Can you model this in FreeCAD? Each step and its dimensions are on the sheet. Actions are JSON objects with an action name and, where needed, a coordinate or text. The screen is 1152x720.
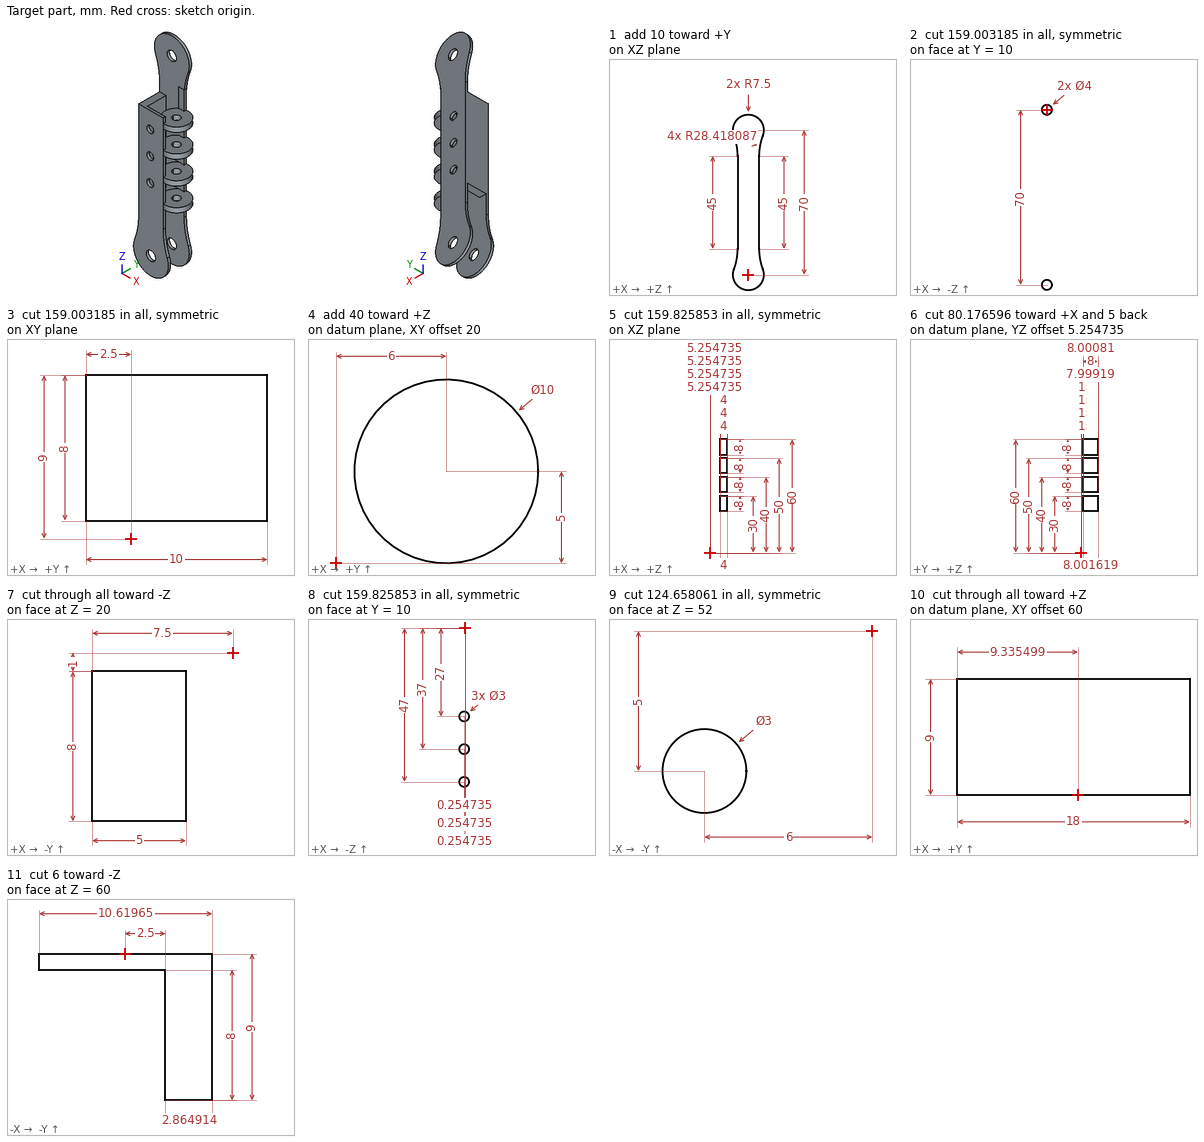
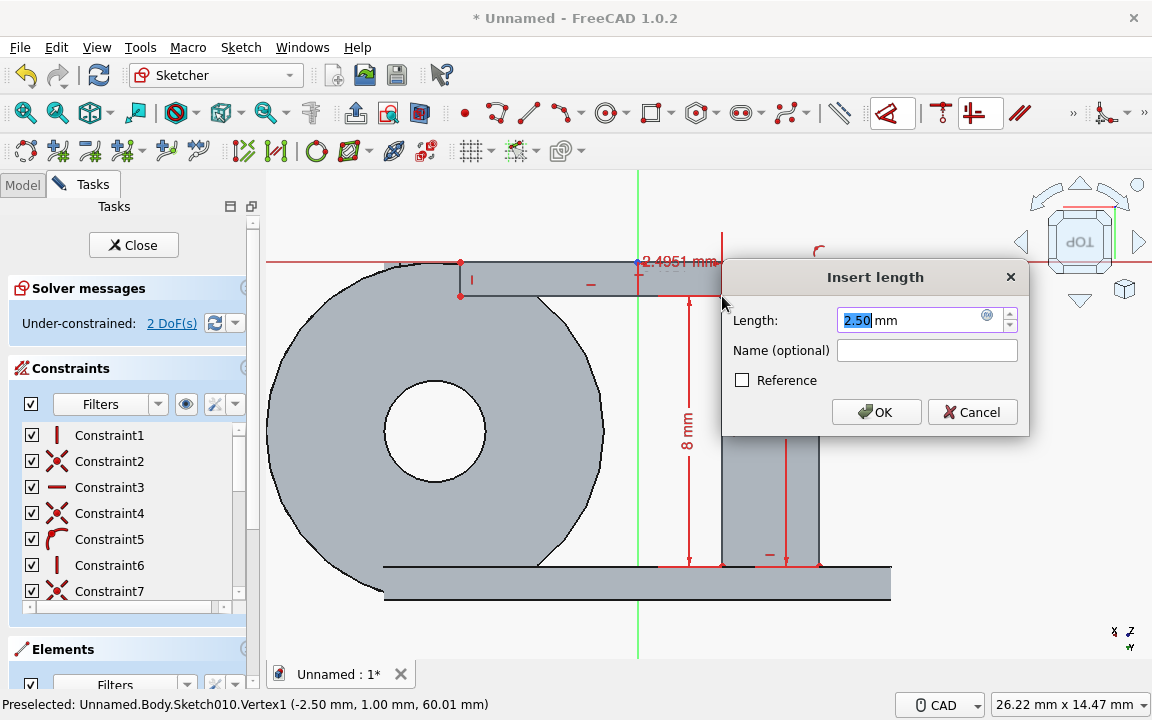
{"action": "type", "text": "2.5"}
{"action": "key", "text": "Return"}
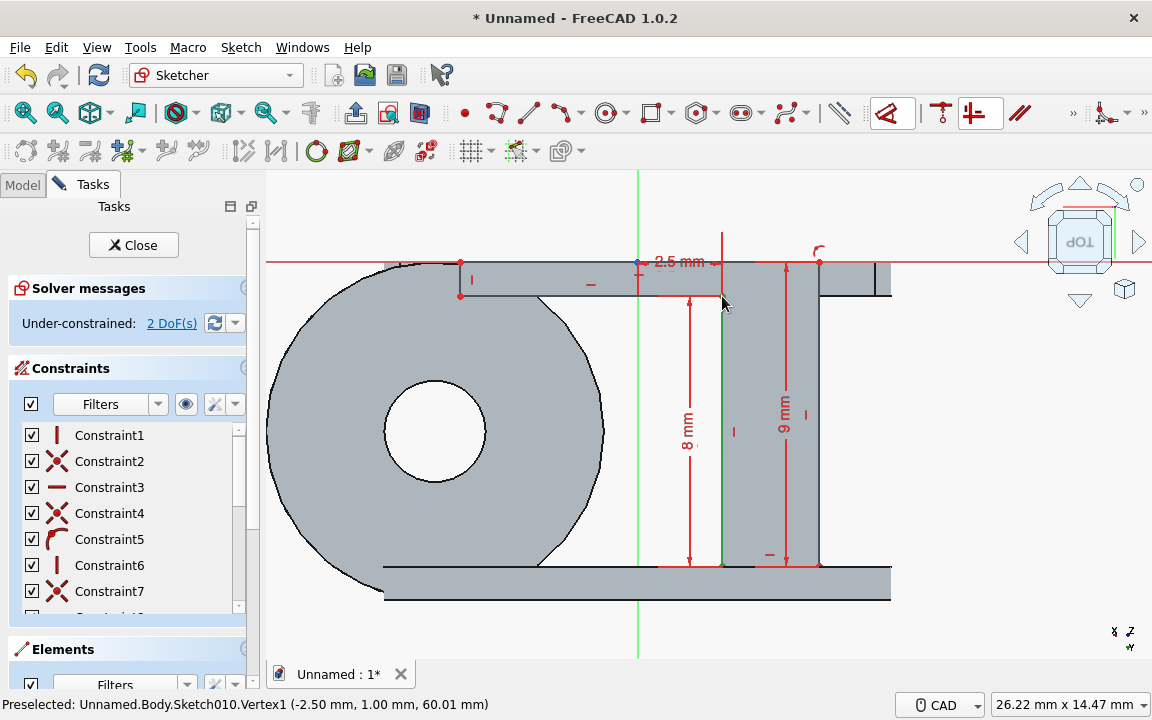
{"action": "left_click", "coordinate": [751, 567]}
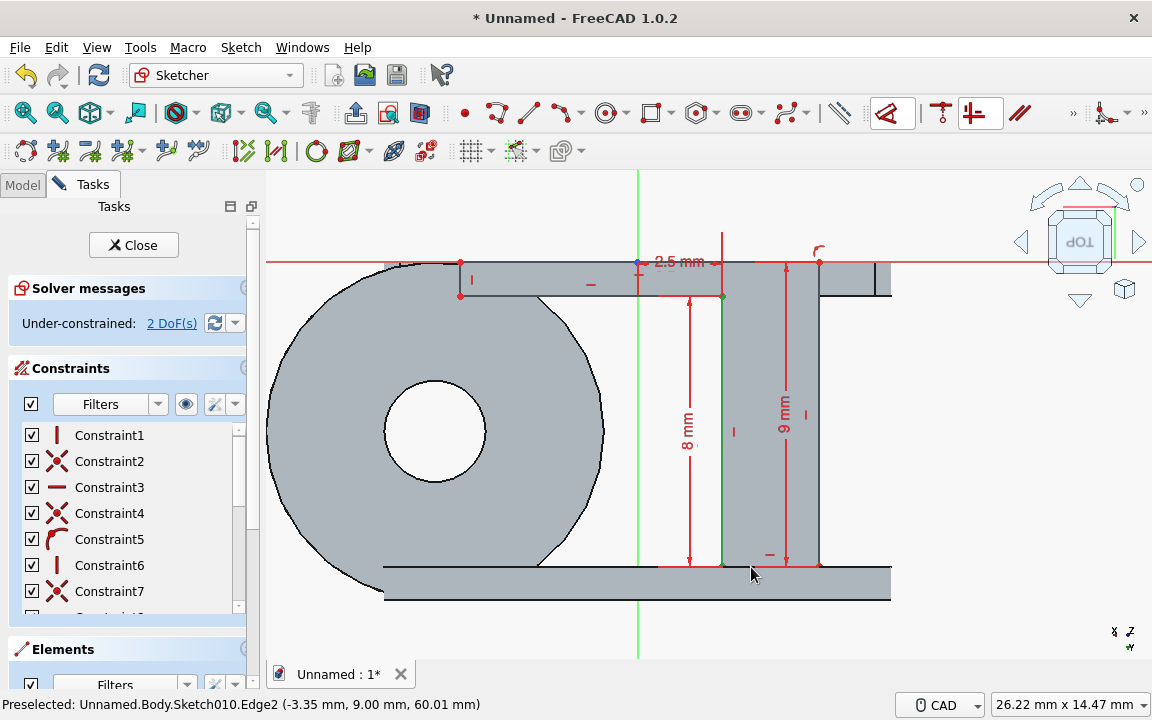
{"action": "key", "text": "l"}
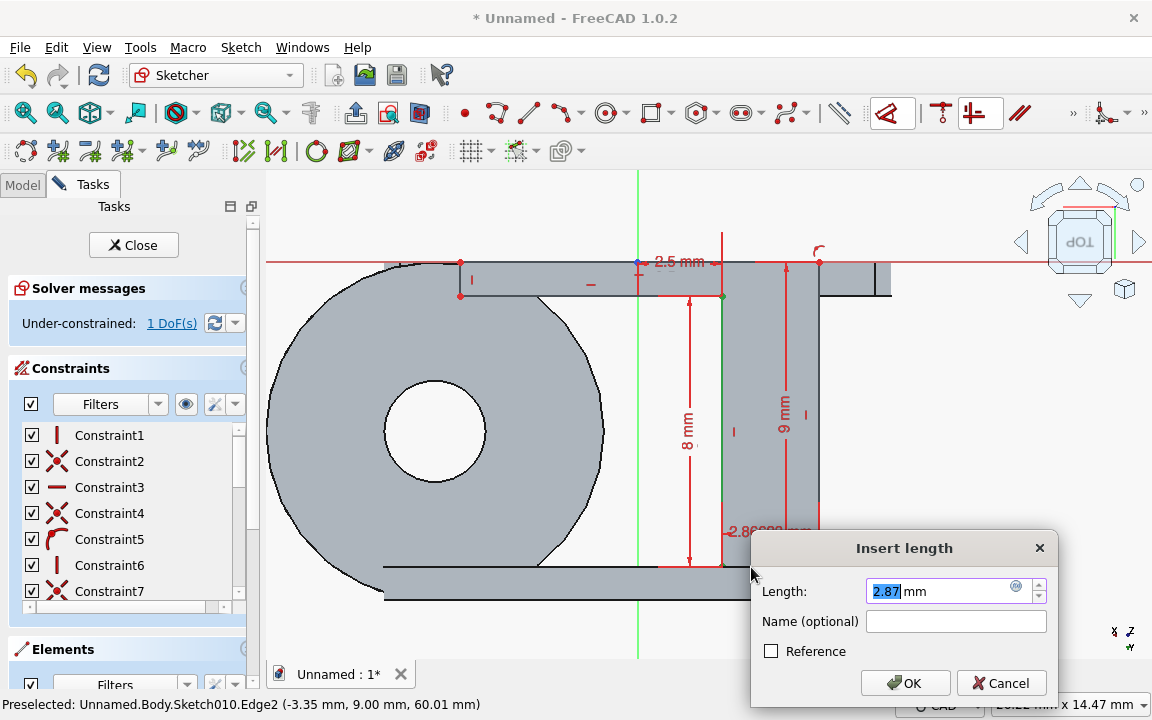
{"action": "type", "text": "2.864914"}
{"action": "key", "text": "Return"}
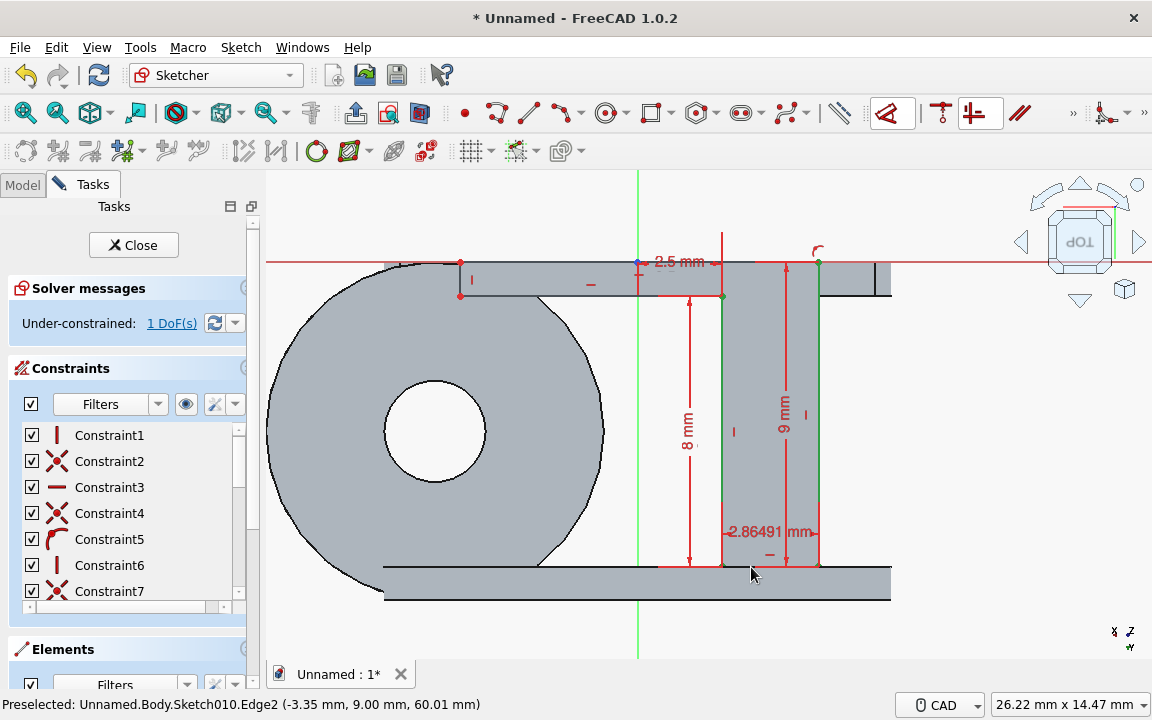
{"action": "left_click", "coordinate": [711, 262]}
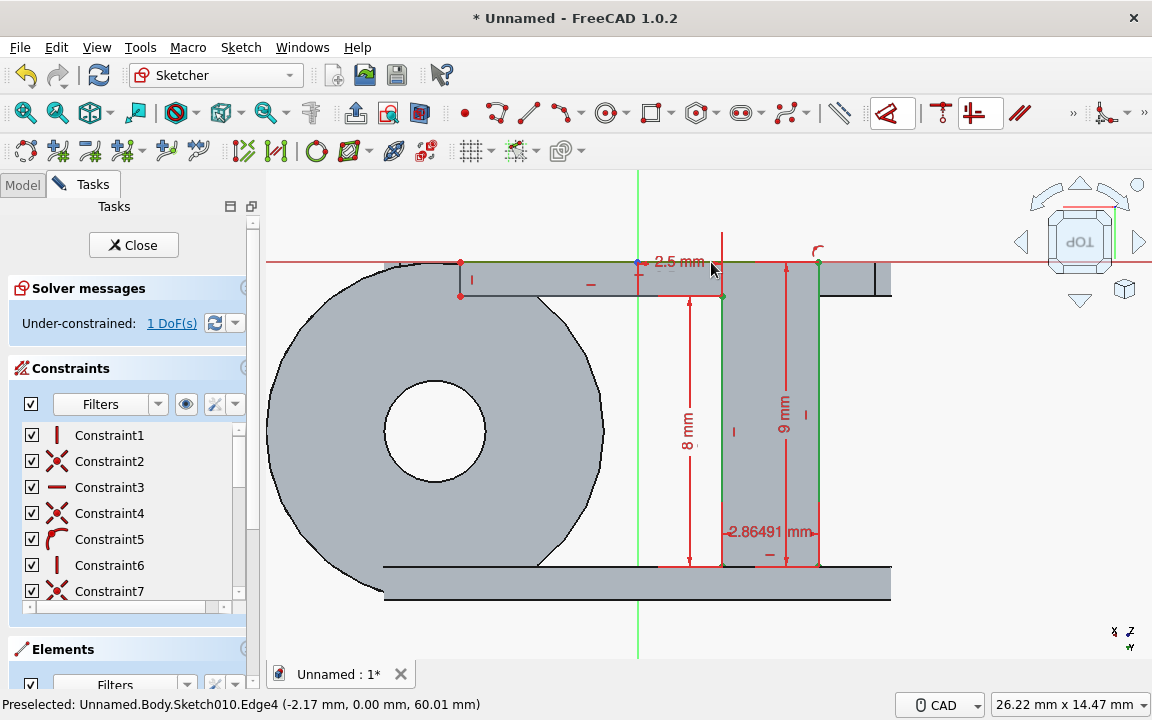
{"action": "left_click", "coordinate": [910, 114]}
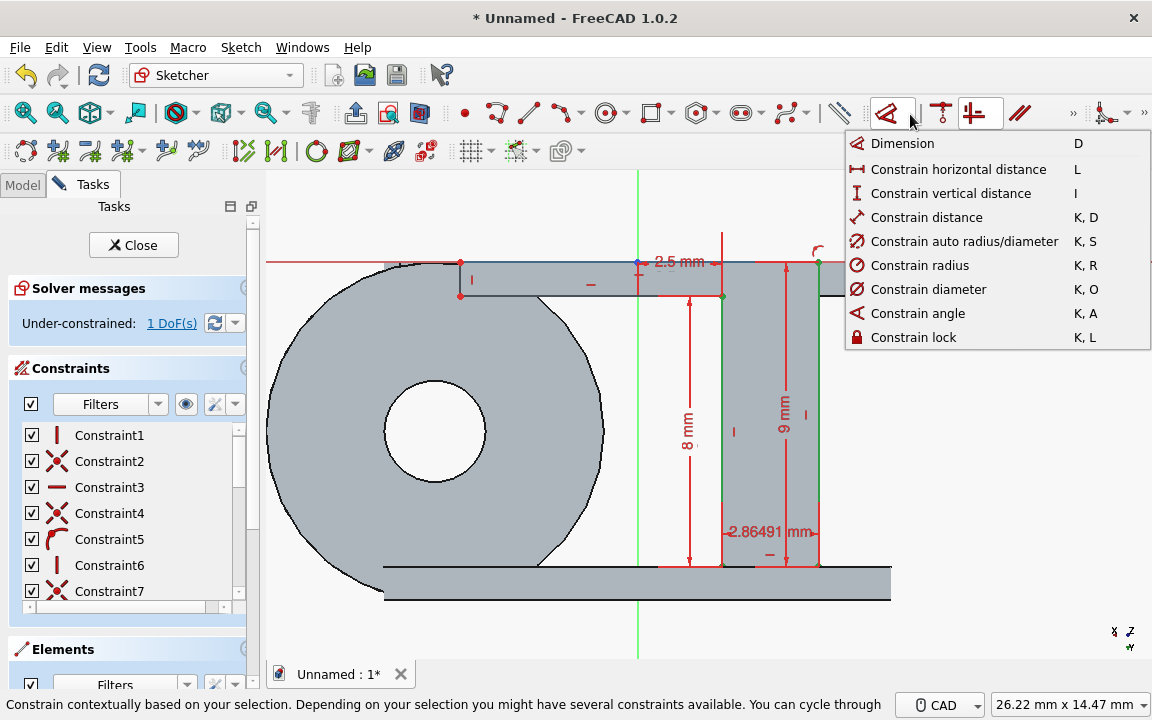
{"action": "left_click", "coordinate": [998, 169]}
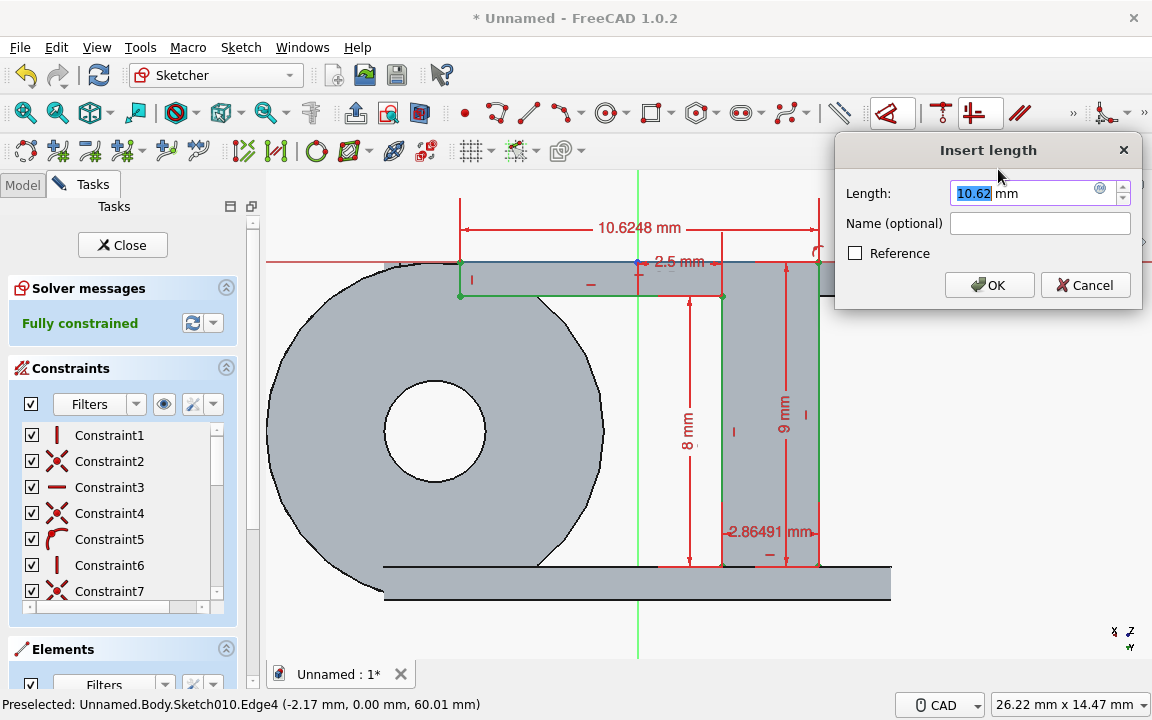
{"action": "type", "text": "10.61965"}
{"action": "key", "text": "Return"}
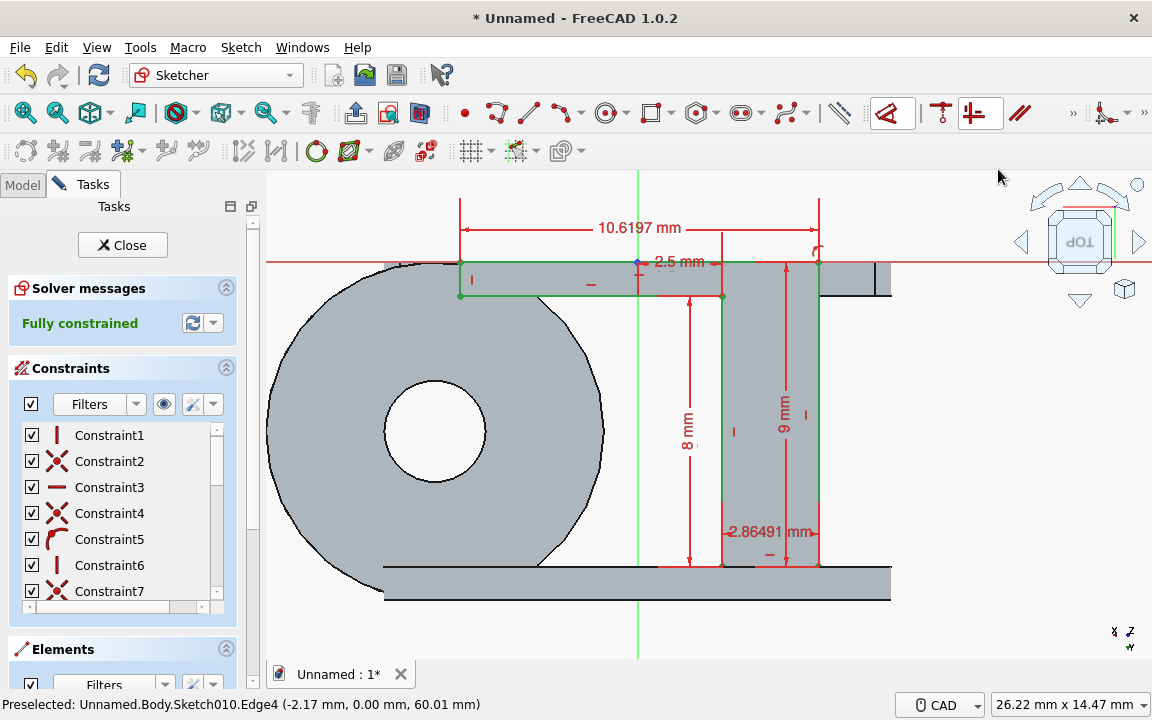
{"action": "left_click", "coordinate": [123, 245]}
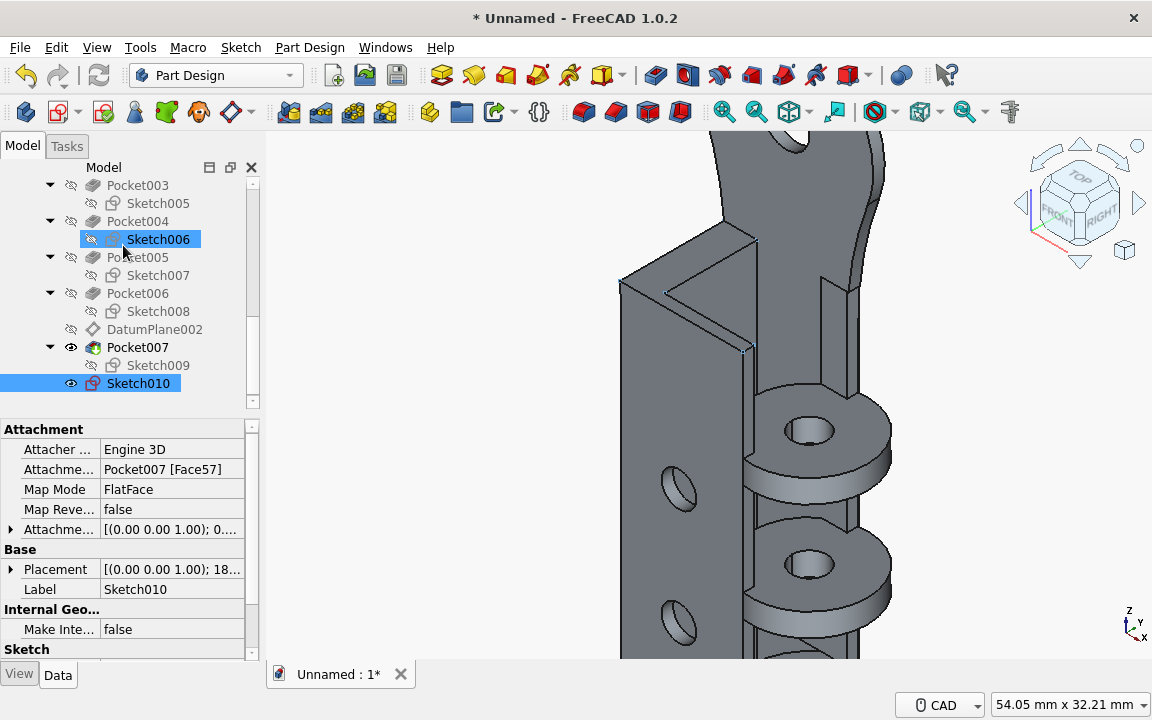
{"action": "left_click", "coordinate": [656, 76]}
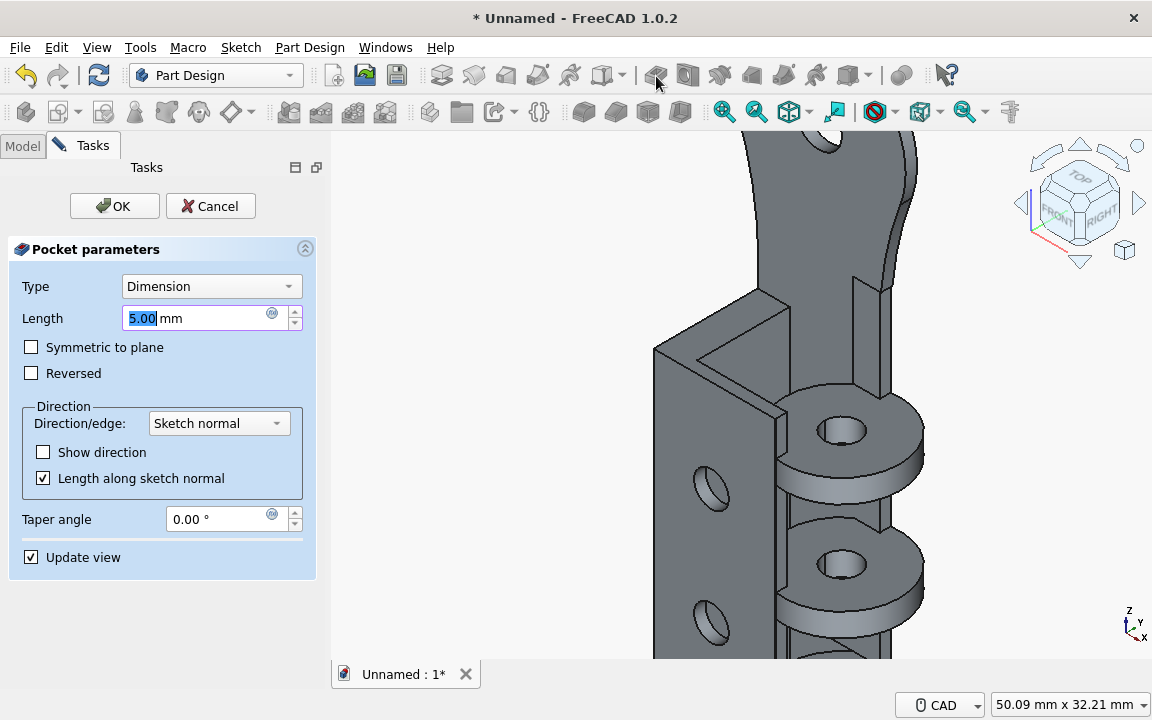
{"action": "type", "text": "6"}
{"action": "key", "text": "Tab"}